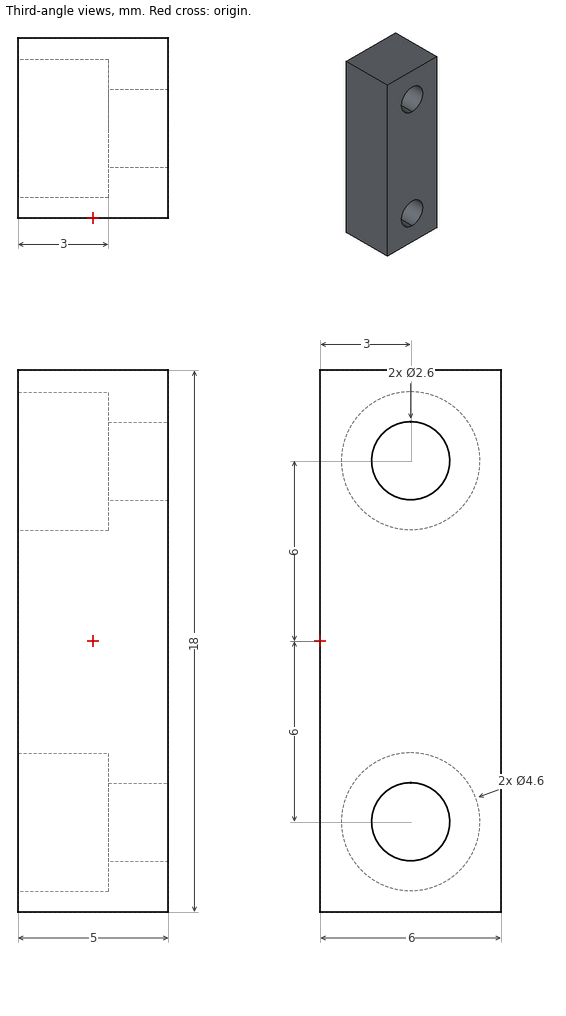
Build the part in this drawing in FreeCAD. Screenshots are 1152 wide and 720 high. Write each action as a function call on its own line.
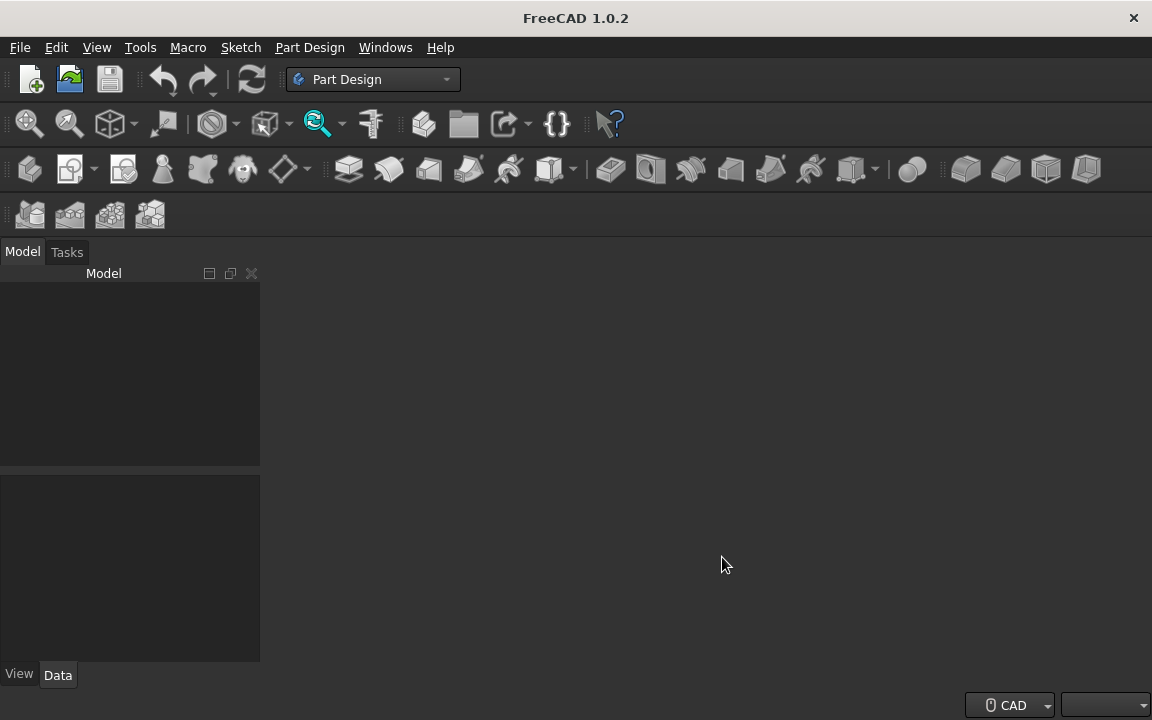
key(ctrl+n)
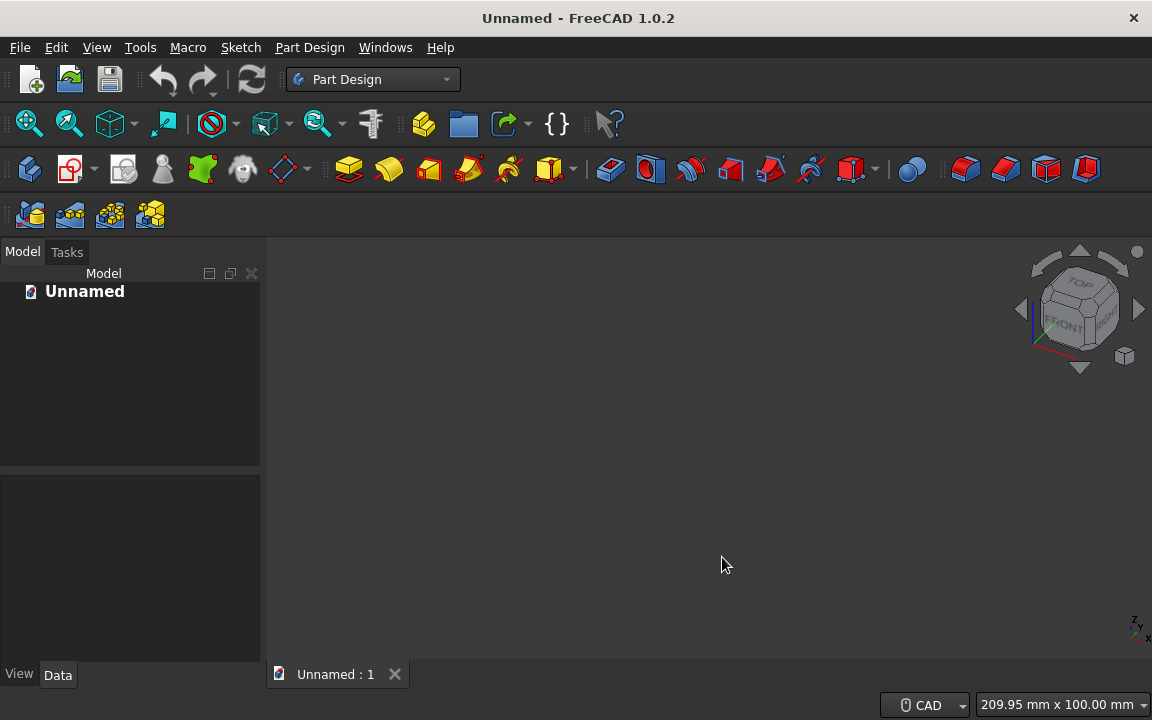
click(70, 170)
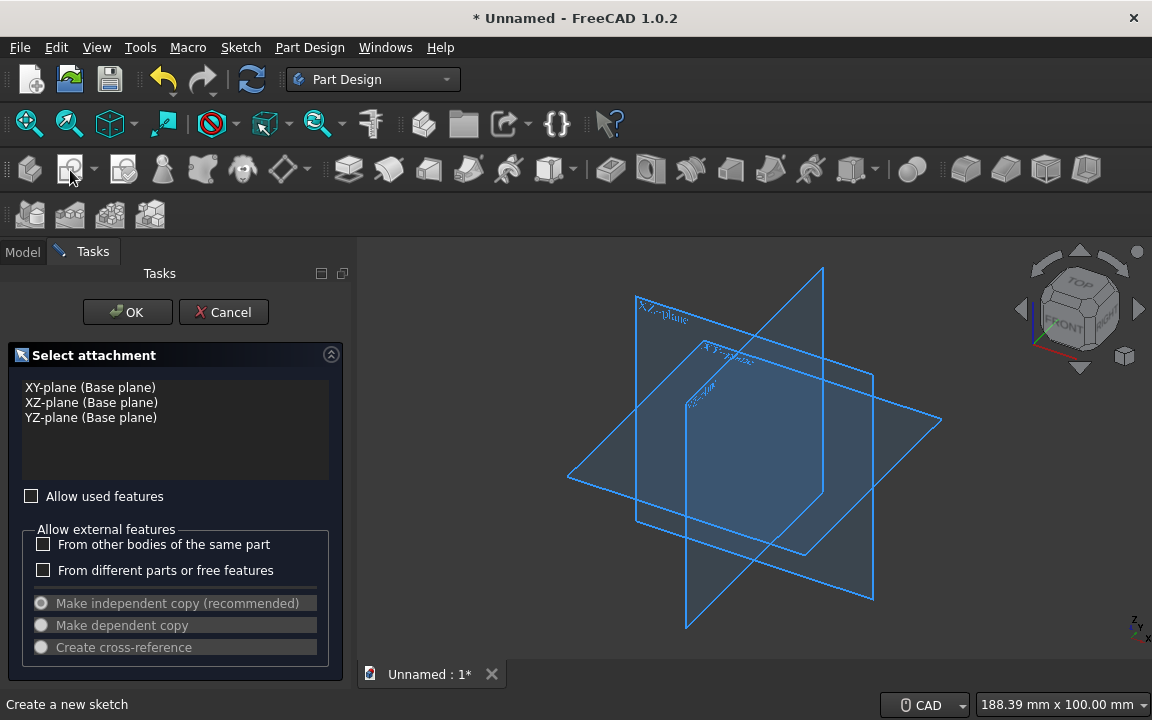
click(82, 402)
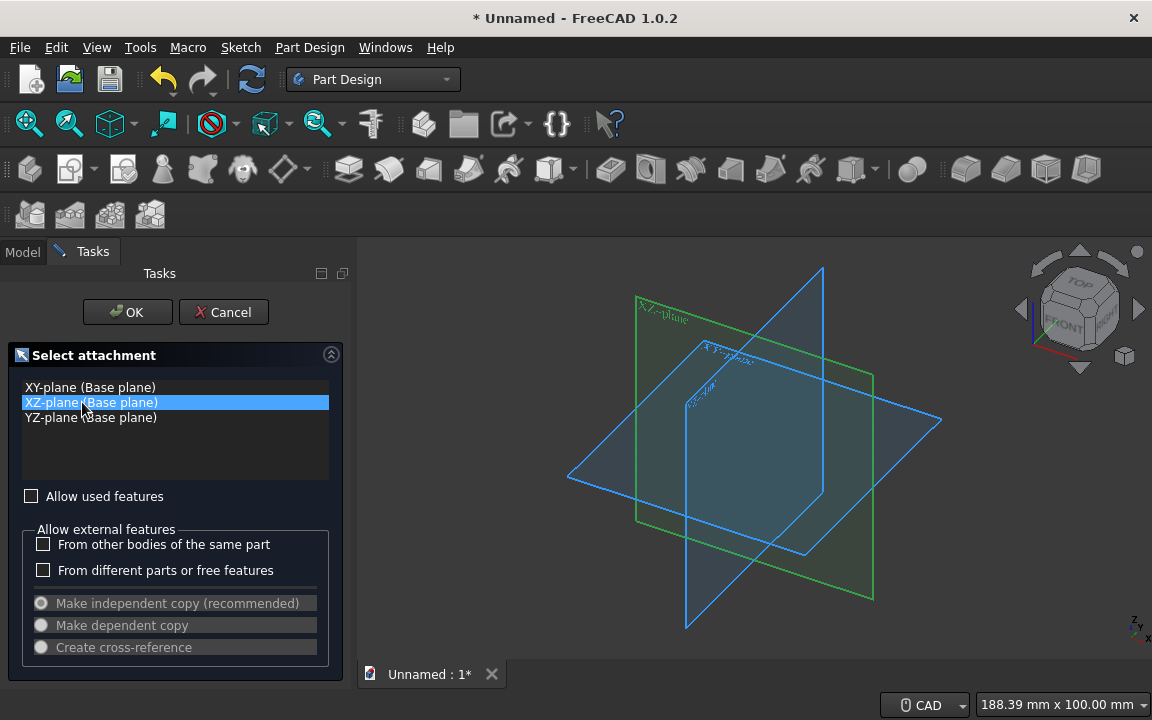
click(128, 312)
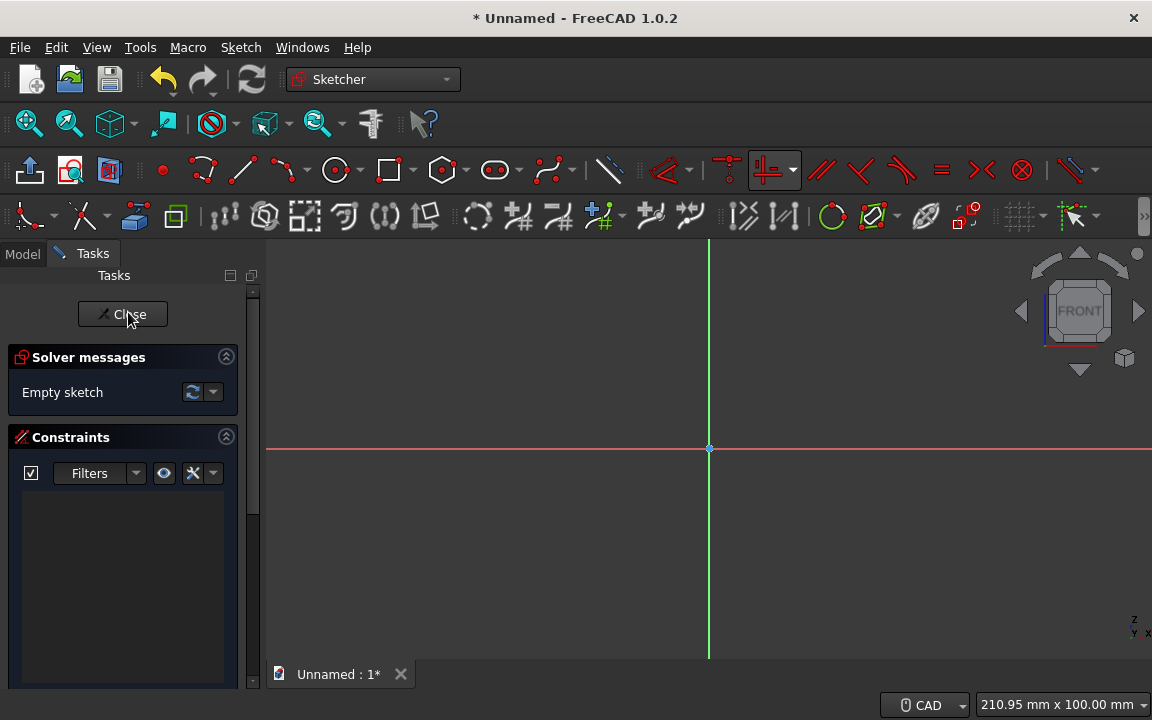
scroll(739, 449, up, 6)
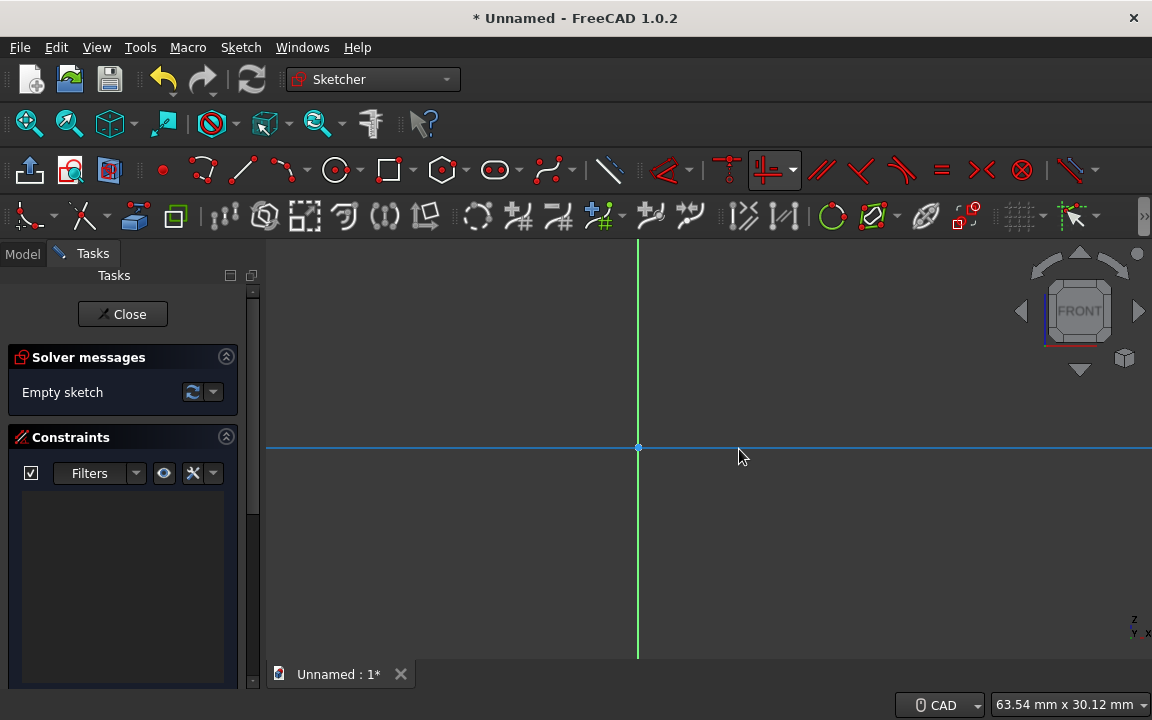
click(416, 170)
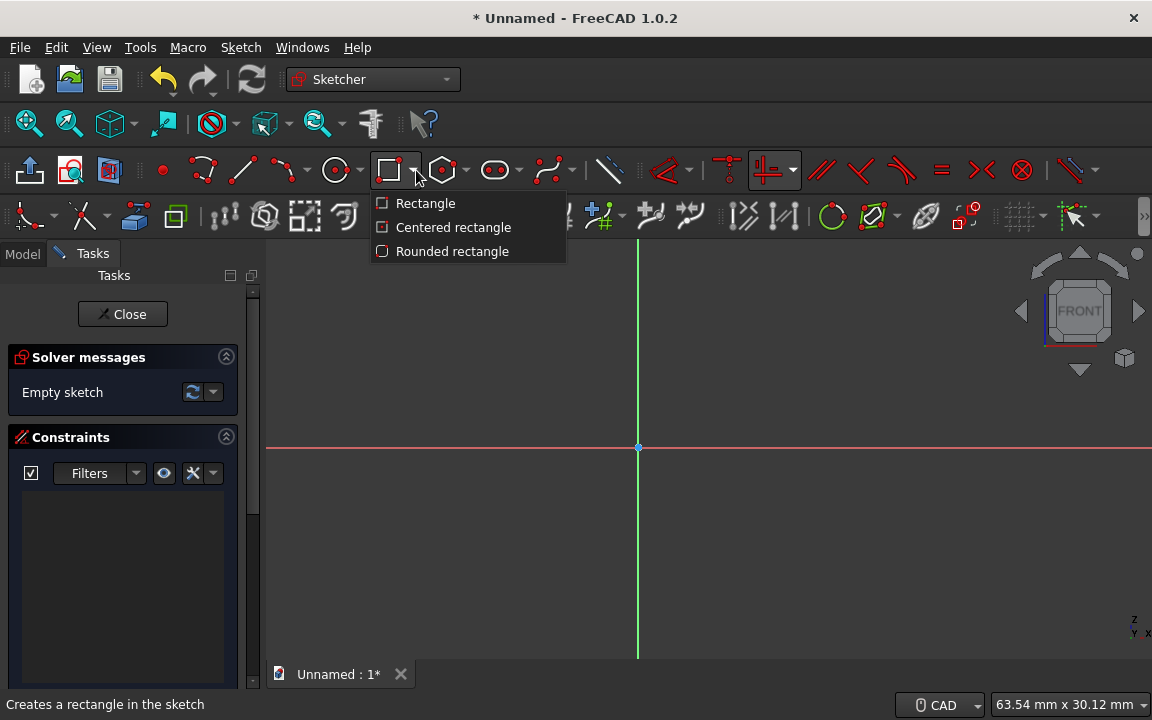
click(468, 227)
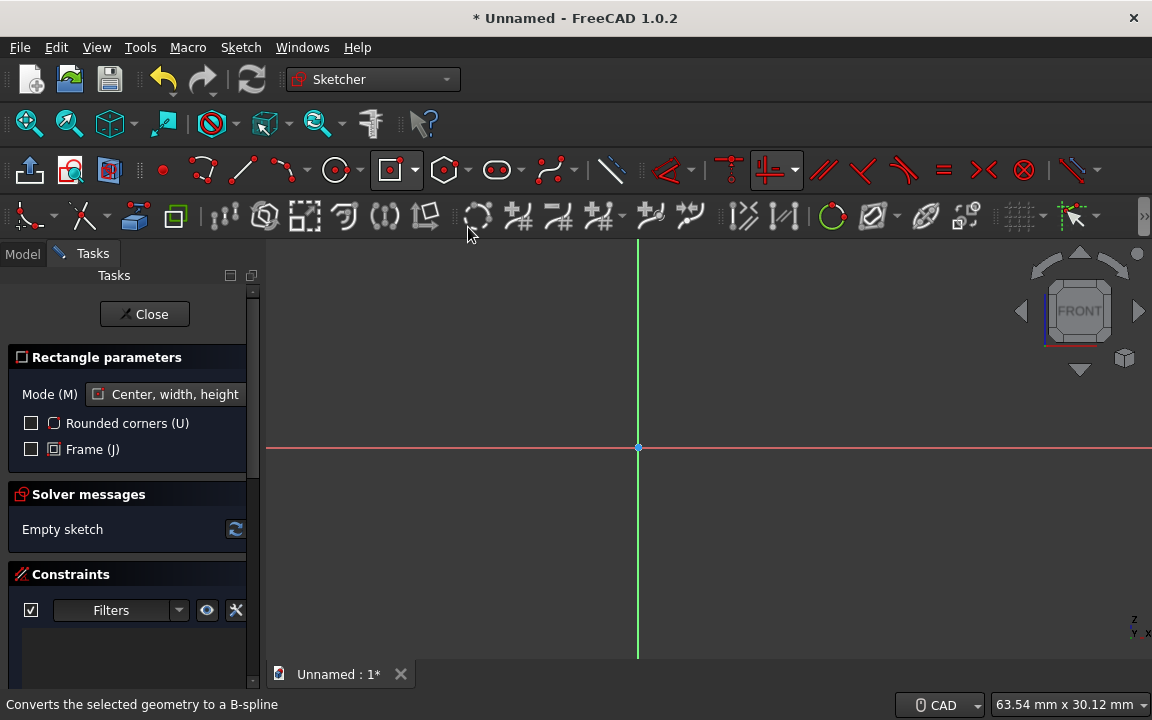
click(638, 448)
click(673, 322)
key(Escape)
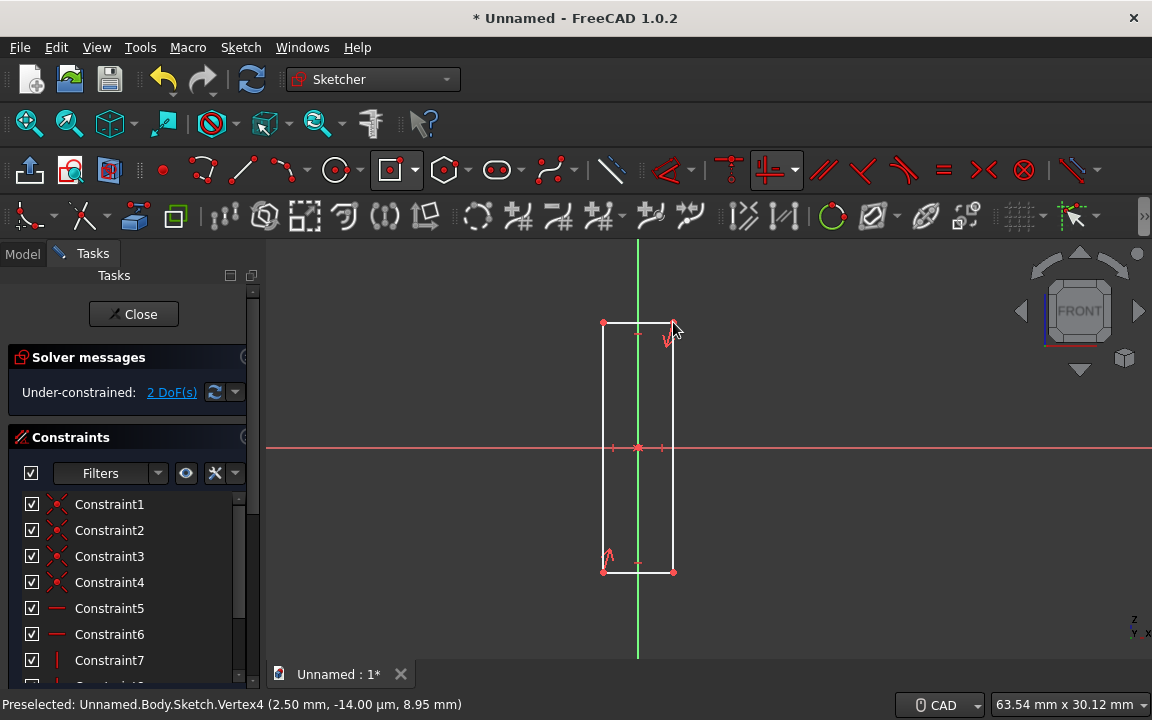
click(666, 170)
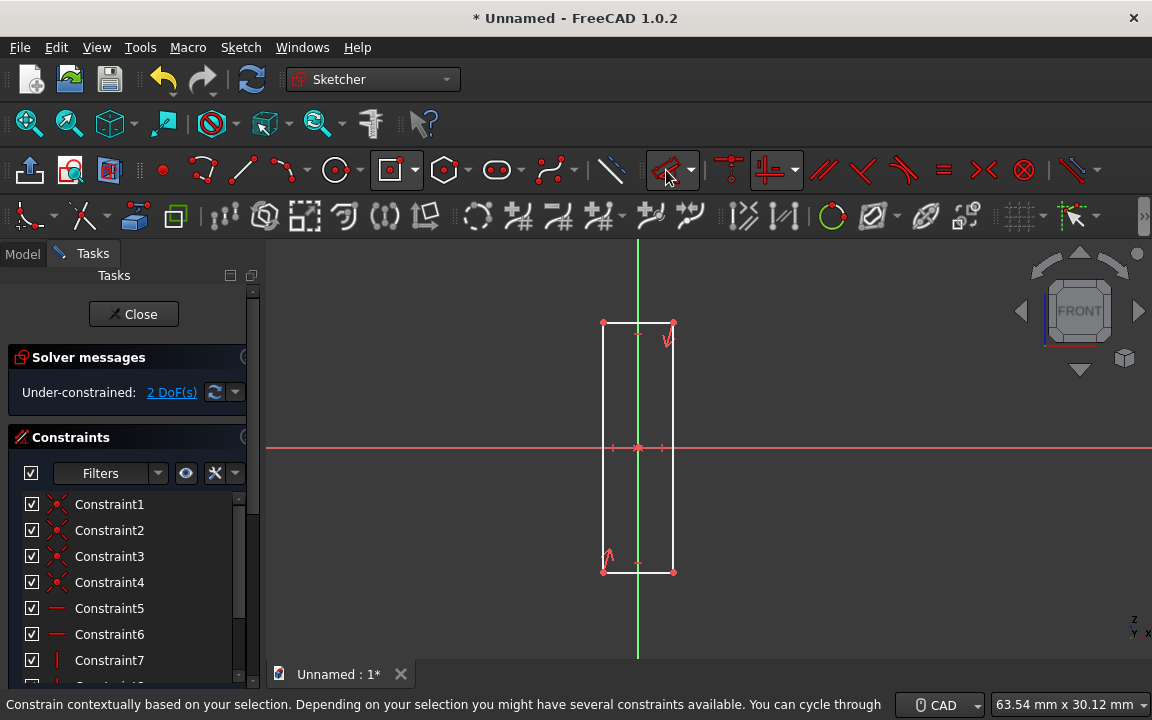
click(624, 573)
click(622, 607)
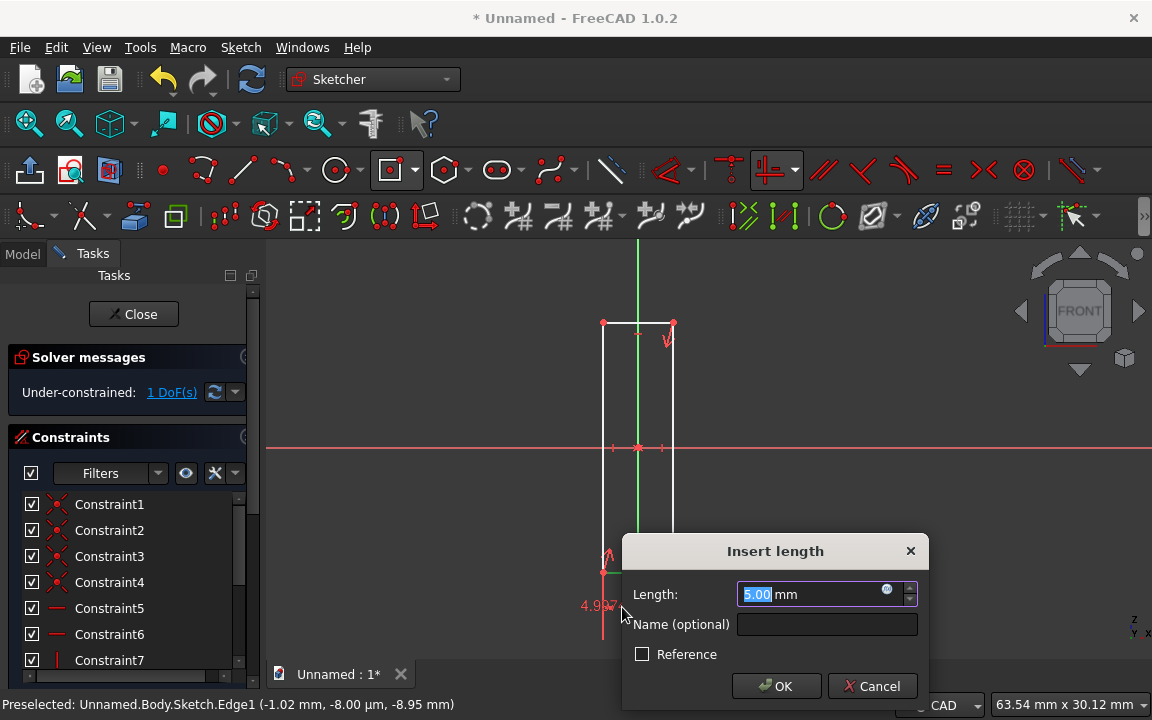
text(5)
key(Return)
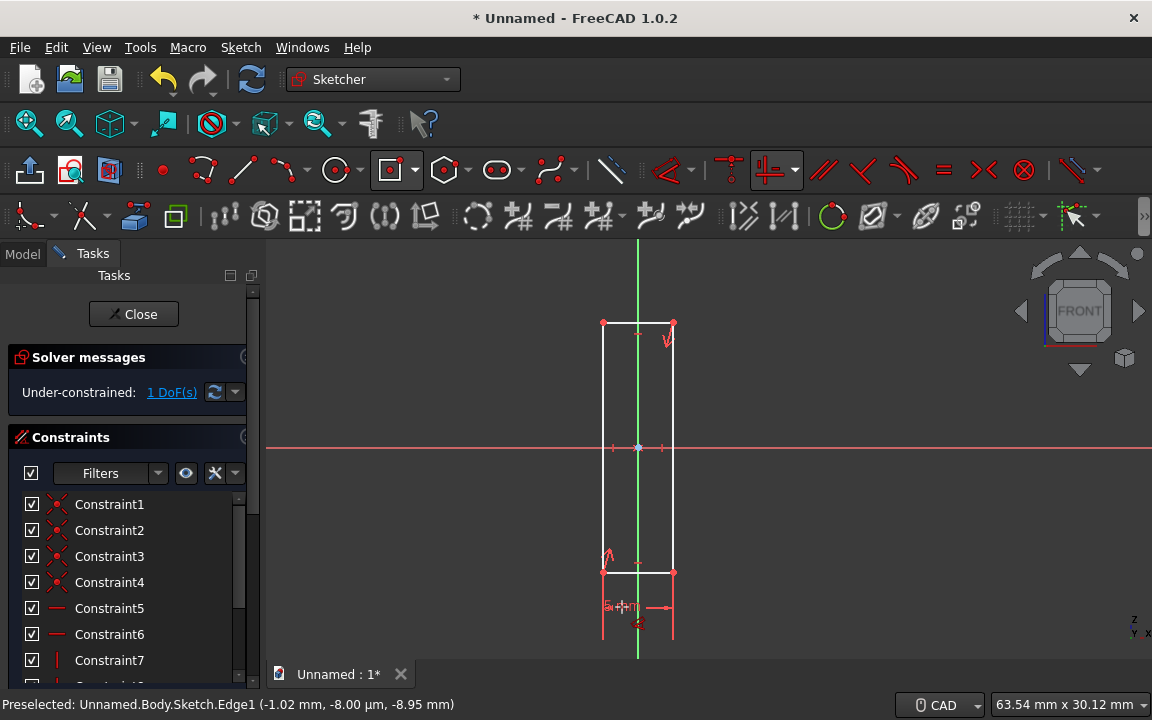
click(673, 498)
click(707, 390)